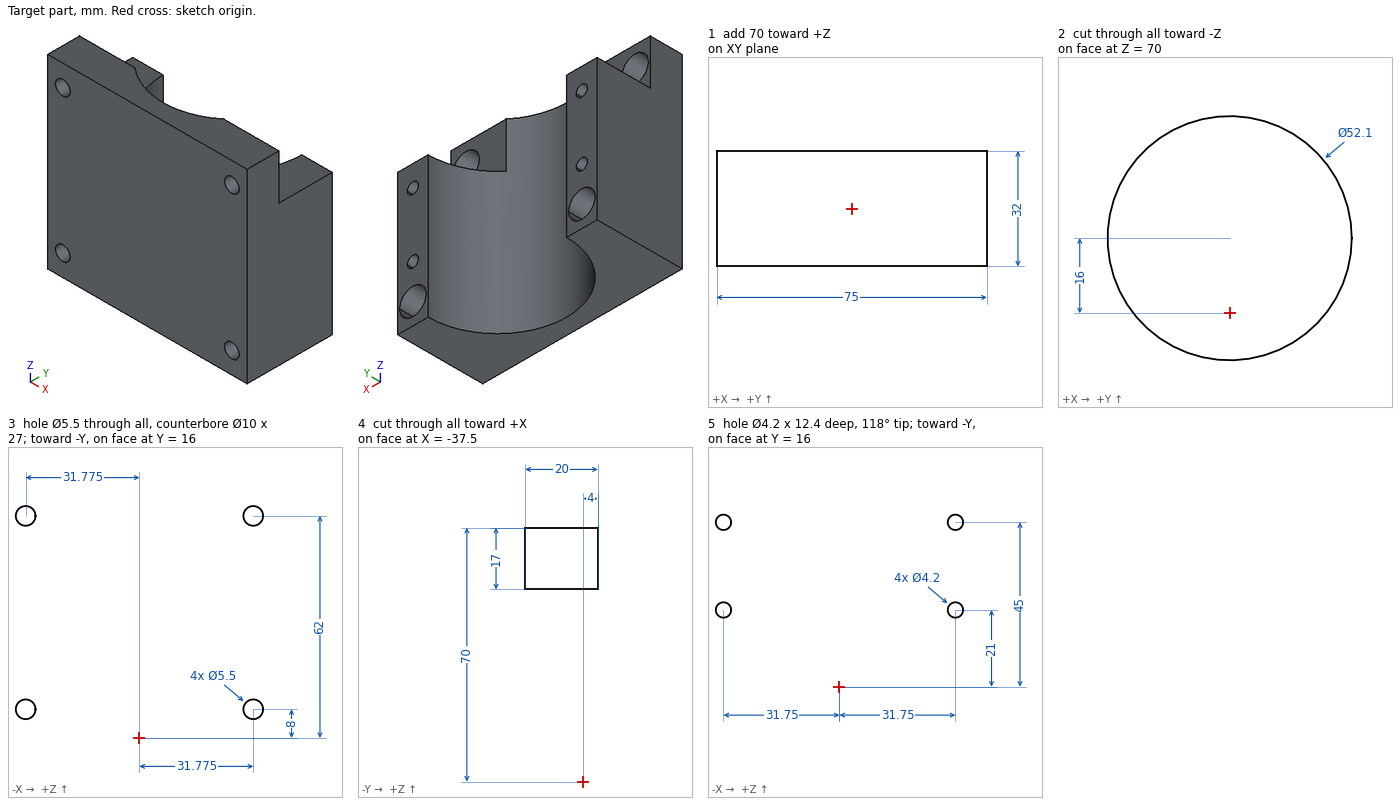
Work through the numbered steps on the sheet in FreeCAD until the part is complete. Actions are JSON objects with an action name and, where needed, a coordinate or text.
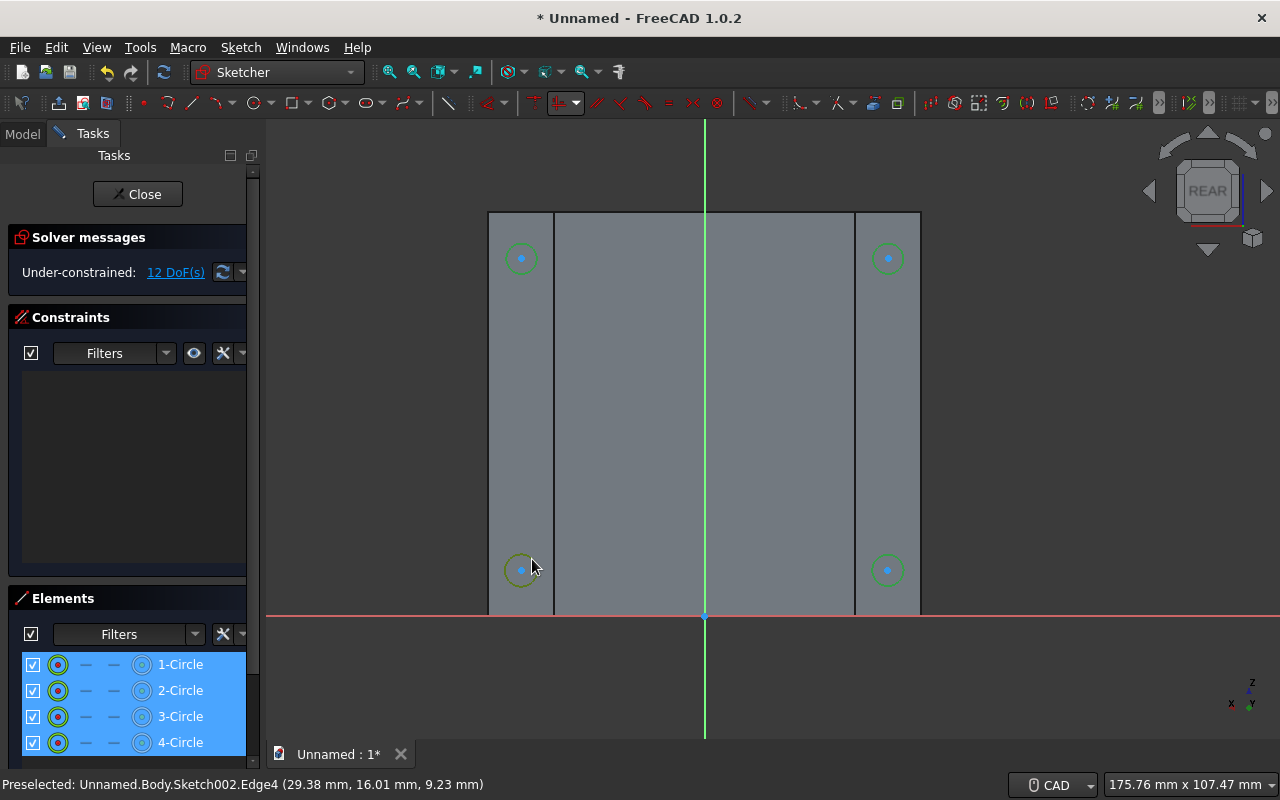
{"action": "left_click", "coordinate": [670, 104]}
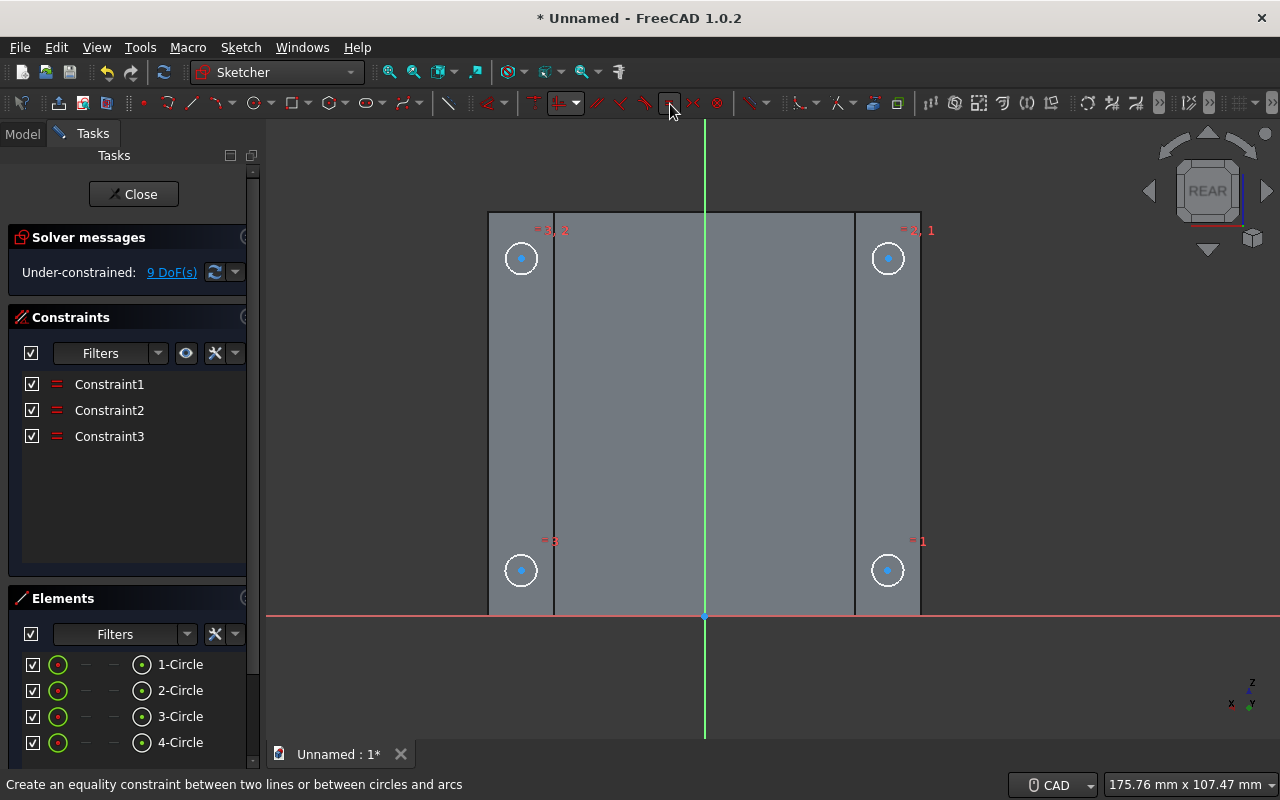
{"action": "left_click", "coordinate": [888, 570]}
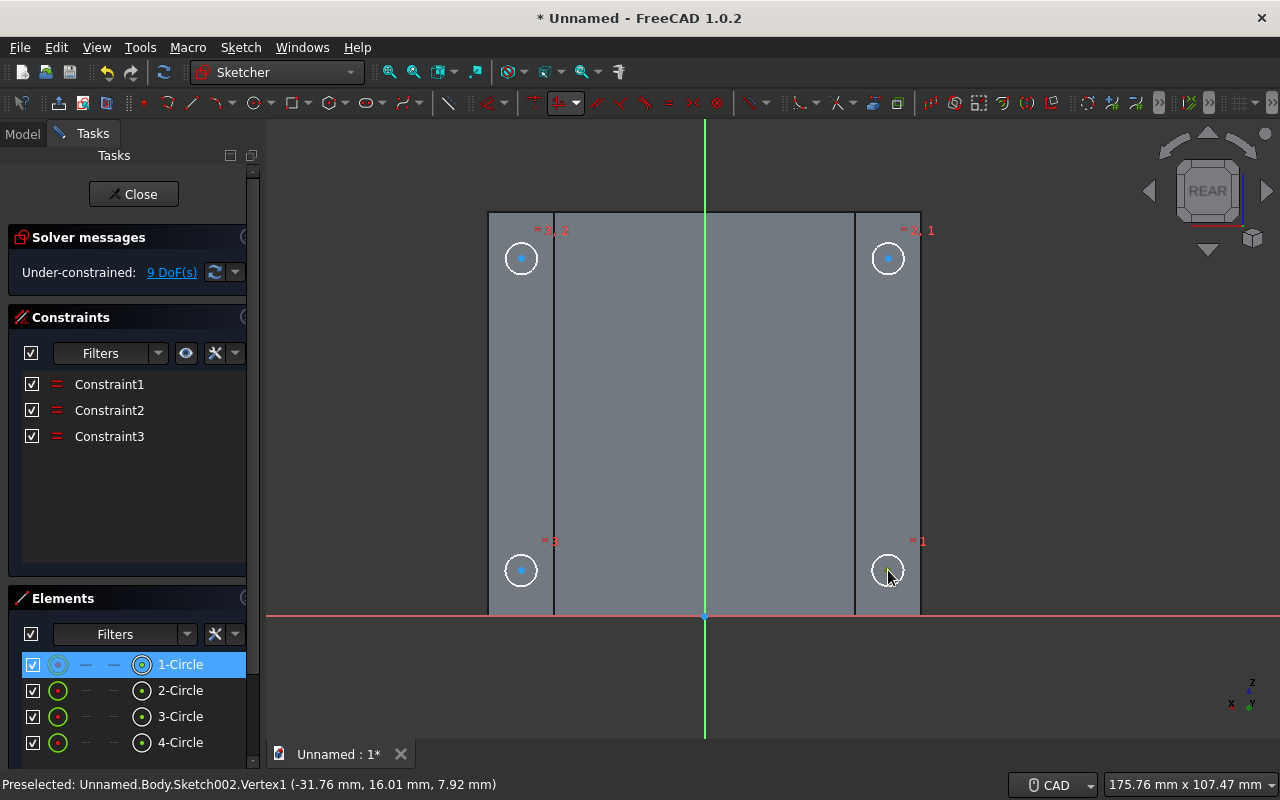
{"action": "left_click", "coordinate": [888, 259]}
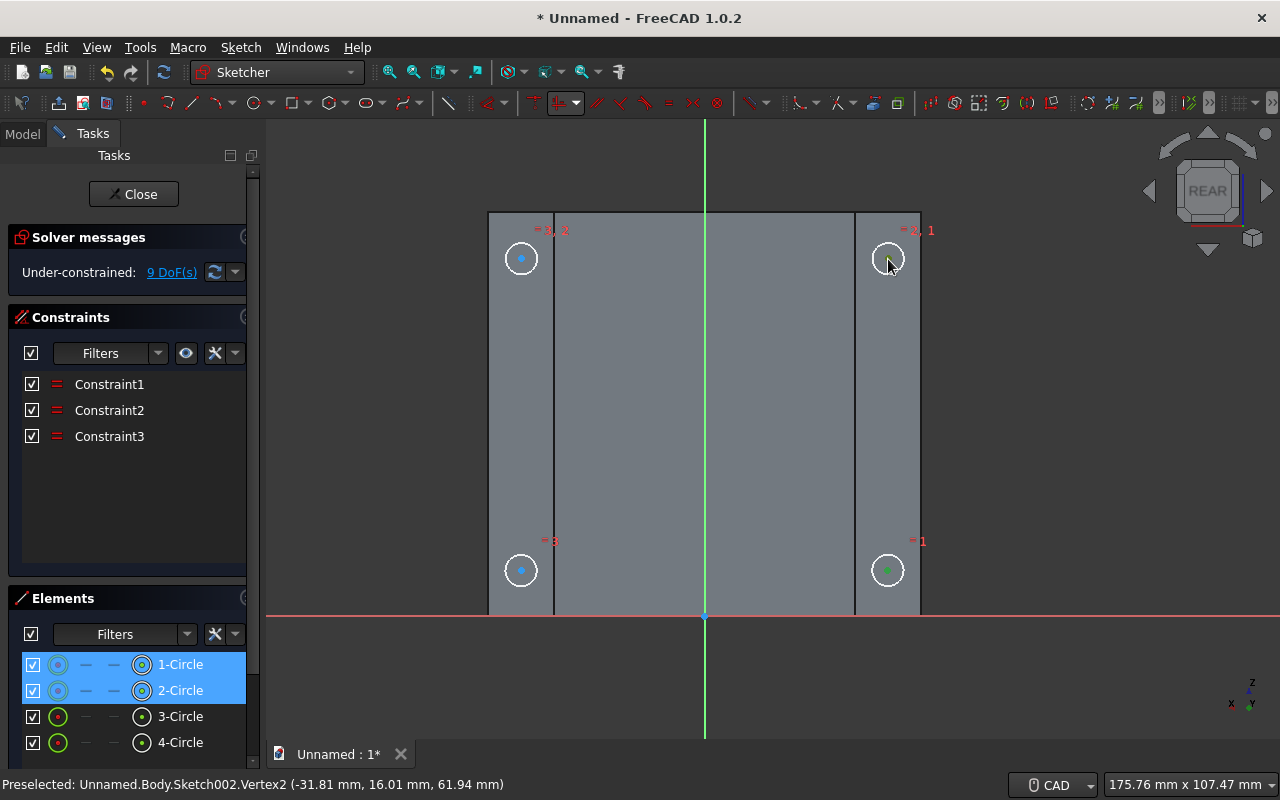
{"action": "left_click", "coordinate": [578, 104]}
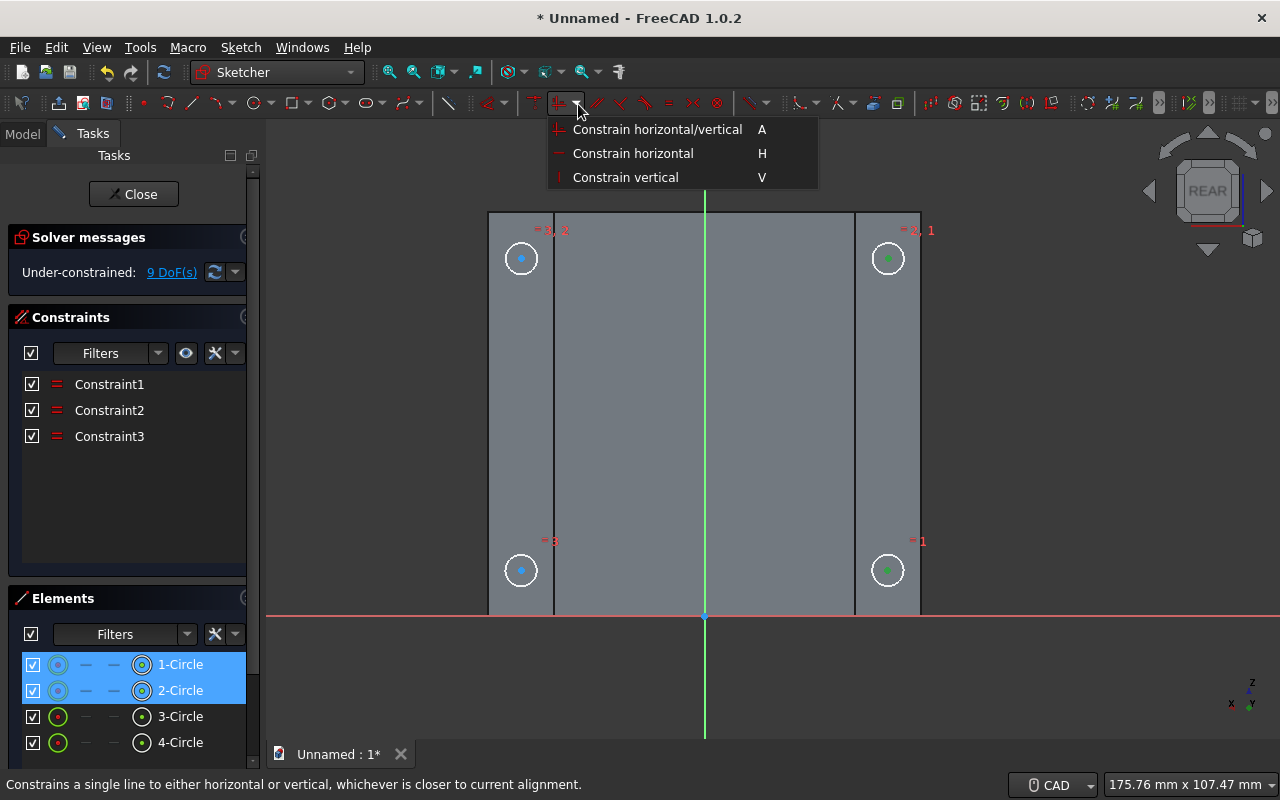
{"action": "left_click", "coordinate": [683, 177]}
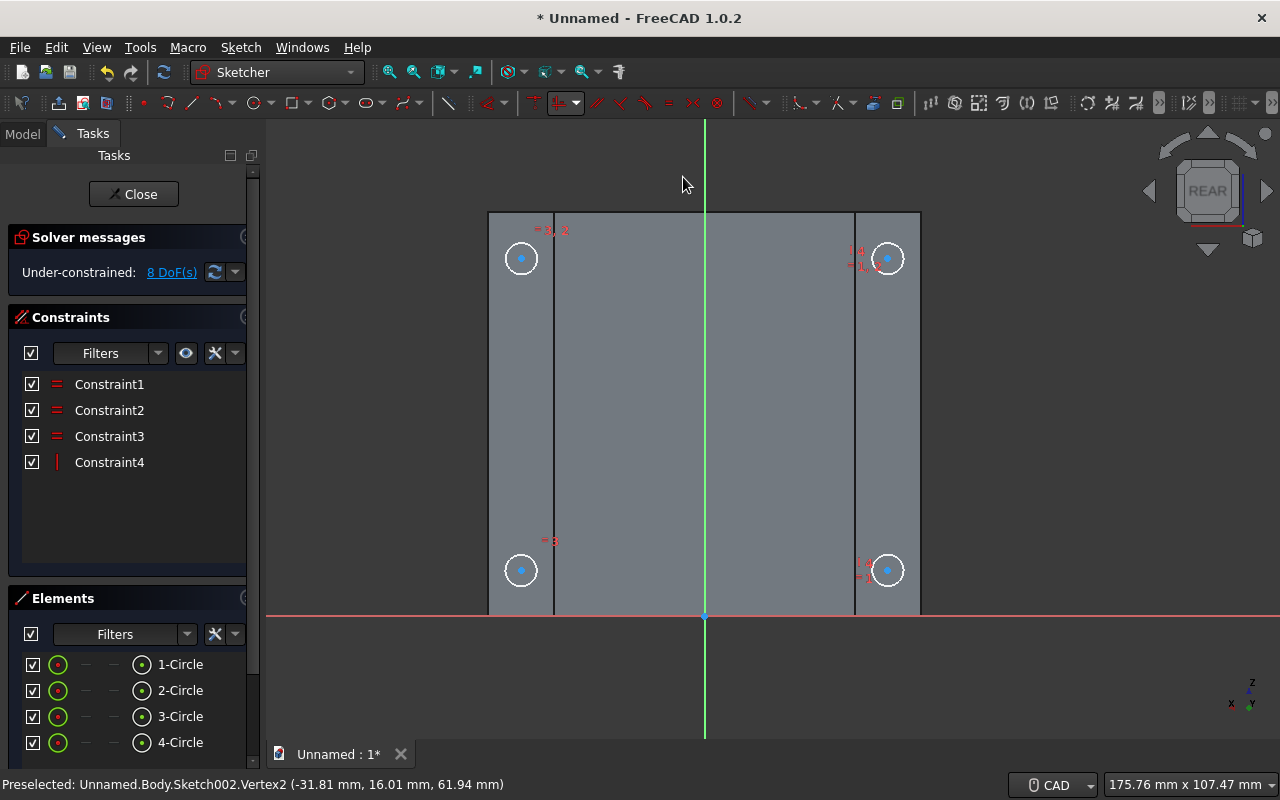
{"action": "left_click", "coordinate": [888, 259]}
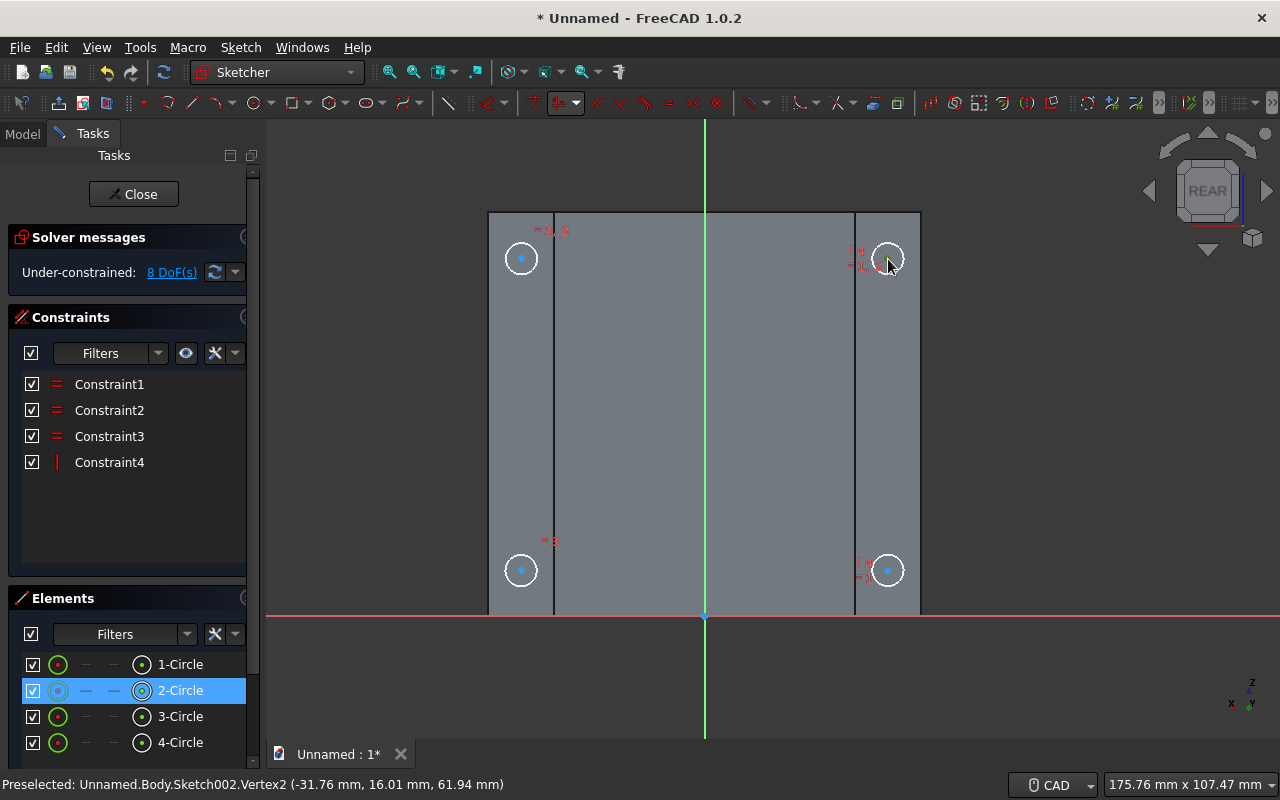
{"action": "left_click", "coordinate": [522, 259]}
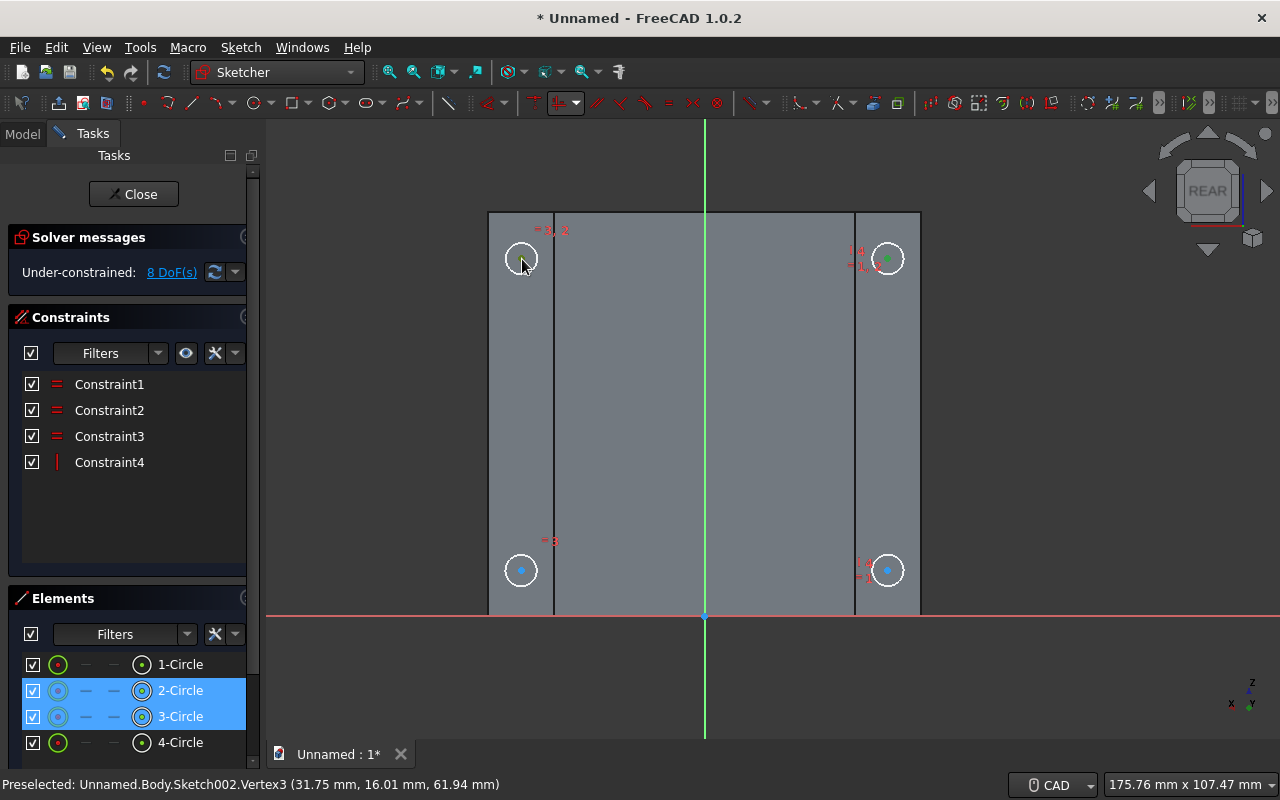
{"action": "left_click", "coordinate": [578, 104]}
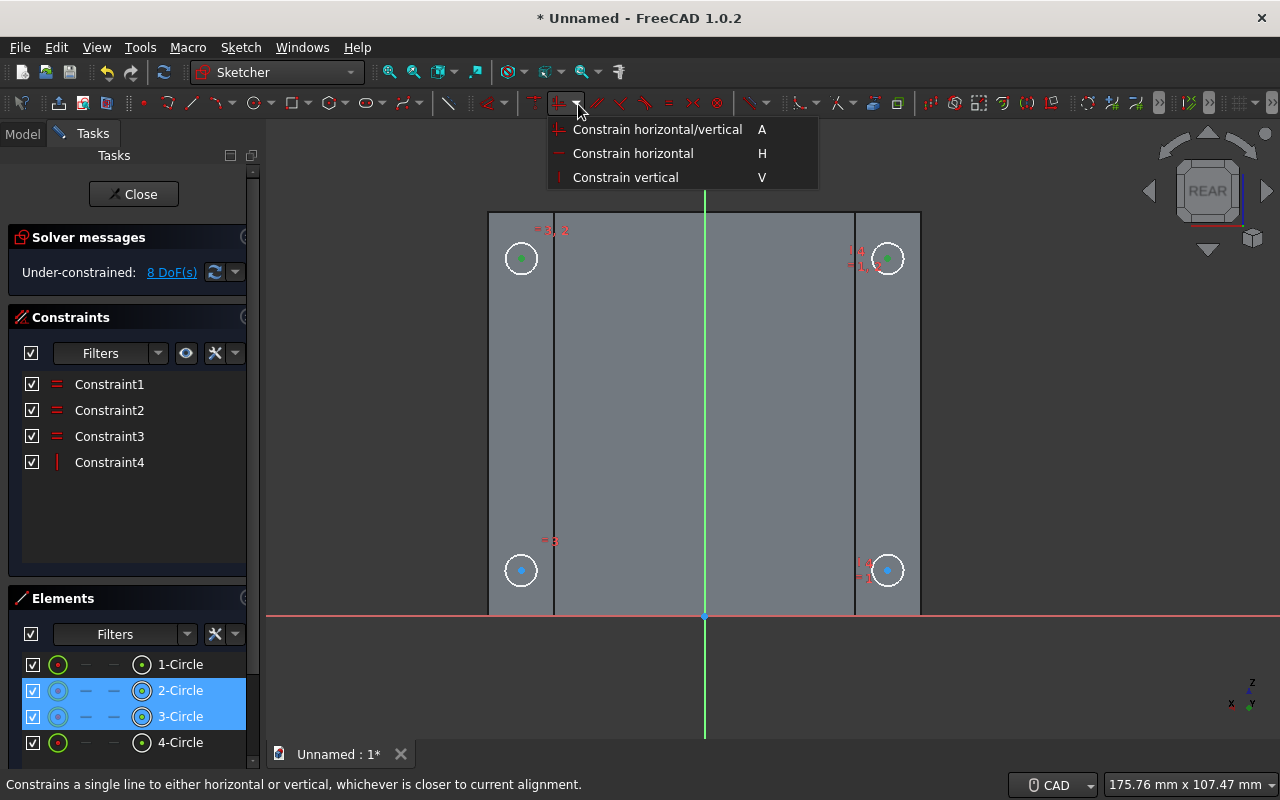
{"action": "left_click", "coordinate": [683, 153]}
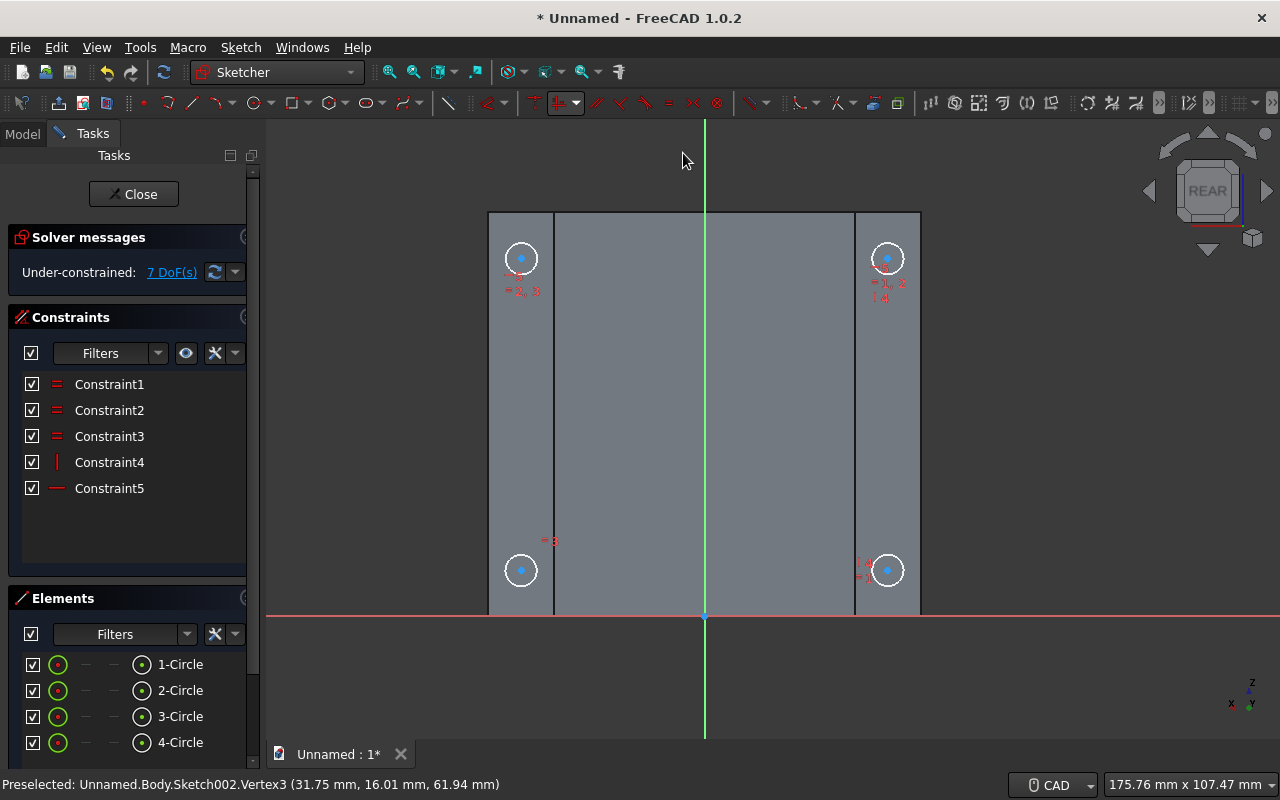
{"action": "left_click", "coordinate": [522, 259]}